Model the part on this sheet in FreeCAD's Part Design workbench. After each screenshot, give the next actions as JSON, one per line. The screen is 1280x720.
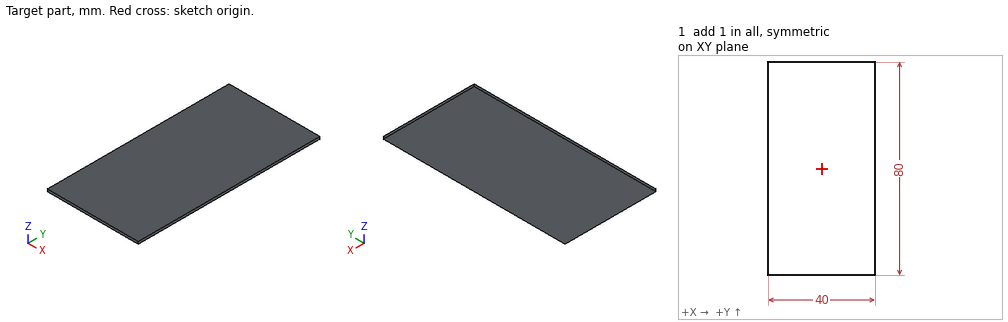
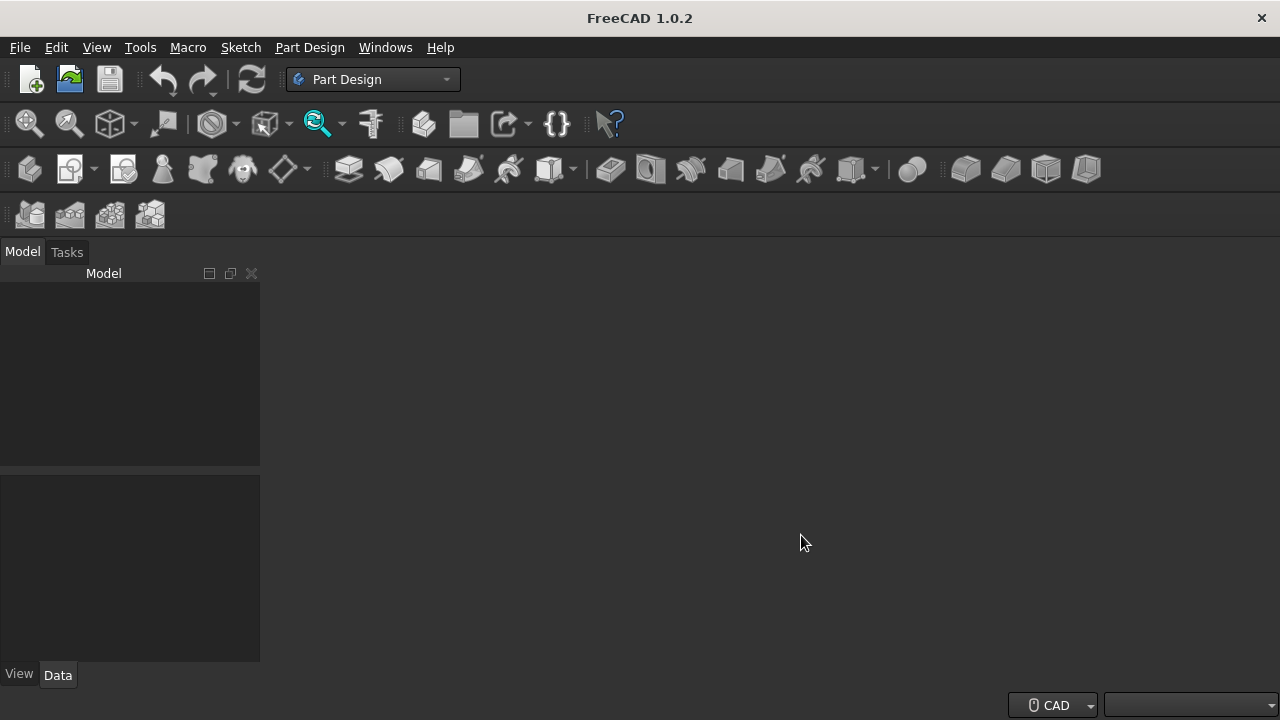
{"action": "left_click", "coordinate": [30, 80]}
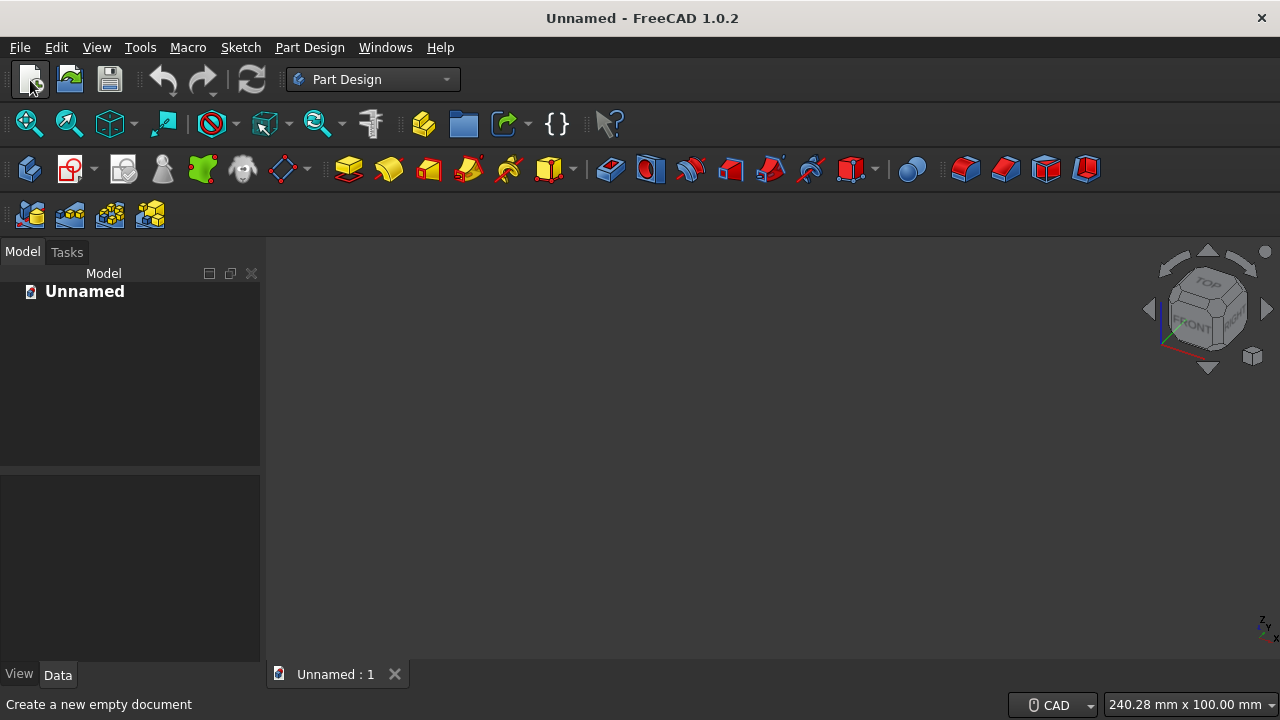
{"action": "left_click", "coordinate": [70, 170]}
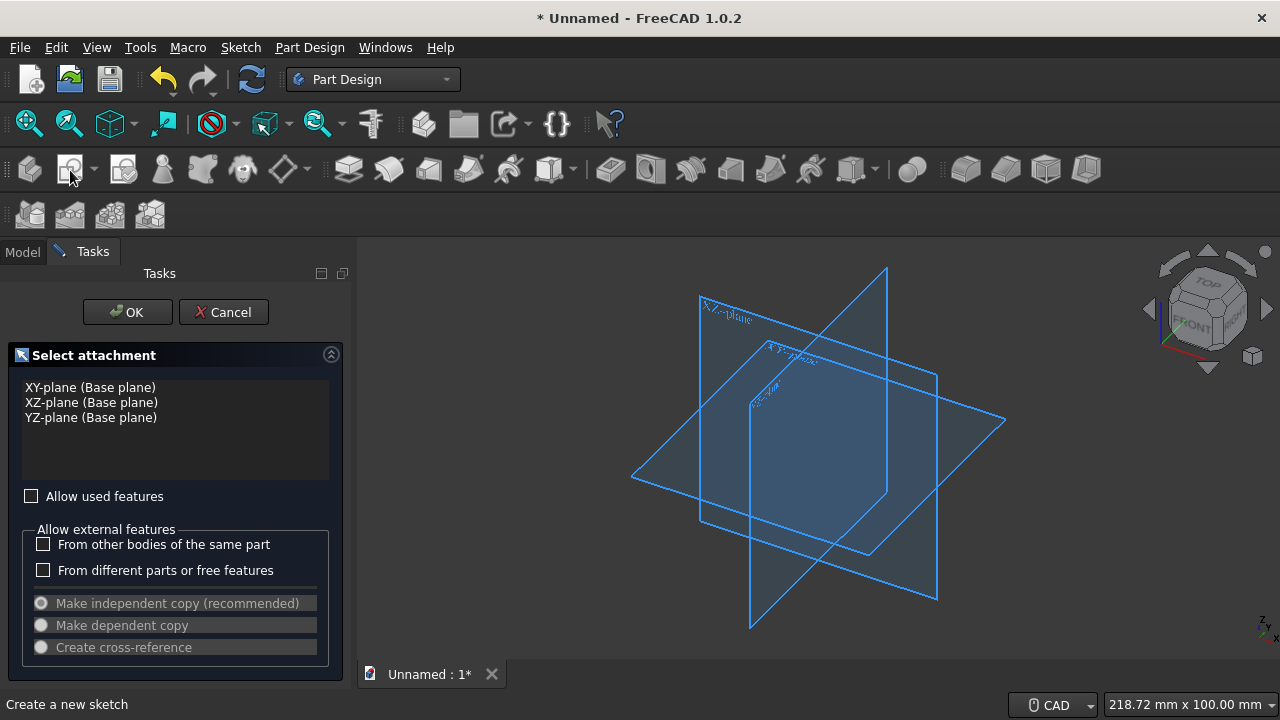
{"action": "left_click", "coordinate": [82, 388]}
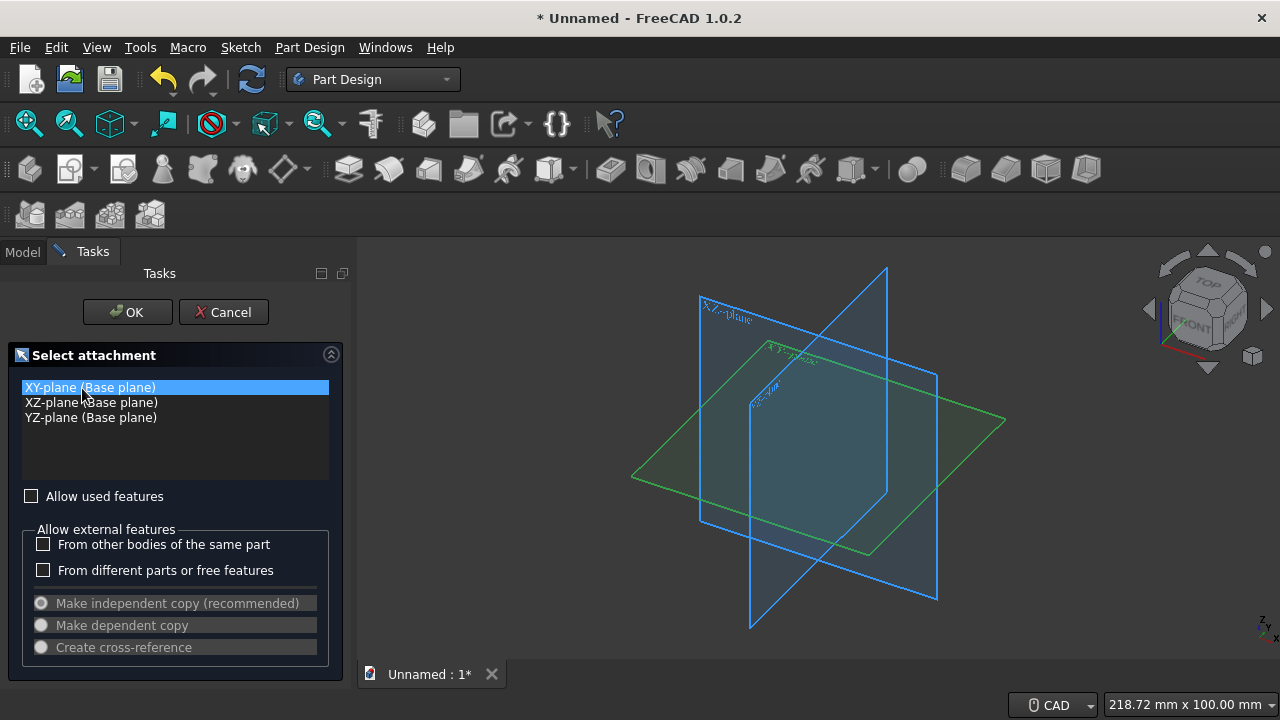
{"action": "left_click", "coordinate": [128, 312]}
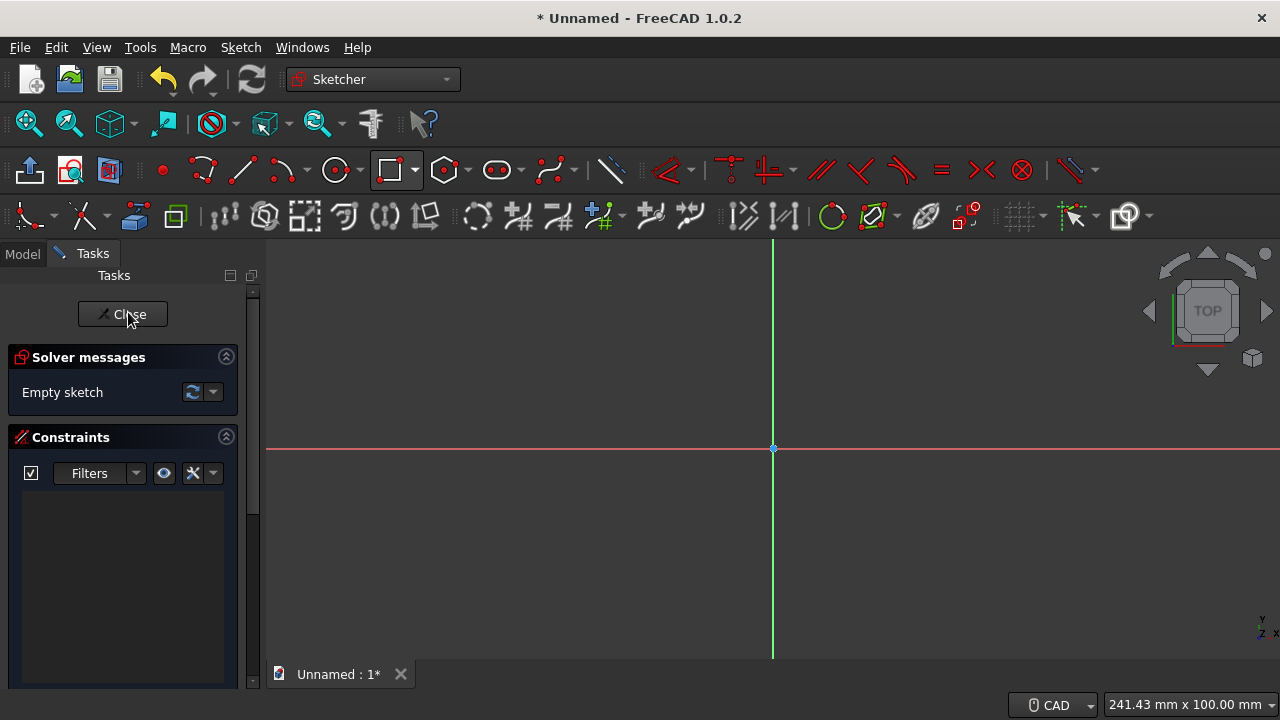
{"action": "scroll", "coordinate": [395, 449], "scroll_direction": "down", "scroll_amount": 1}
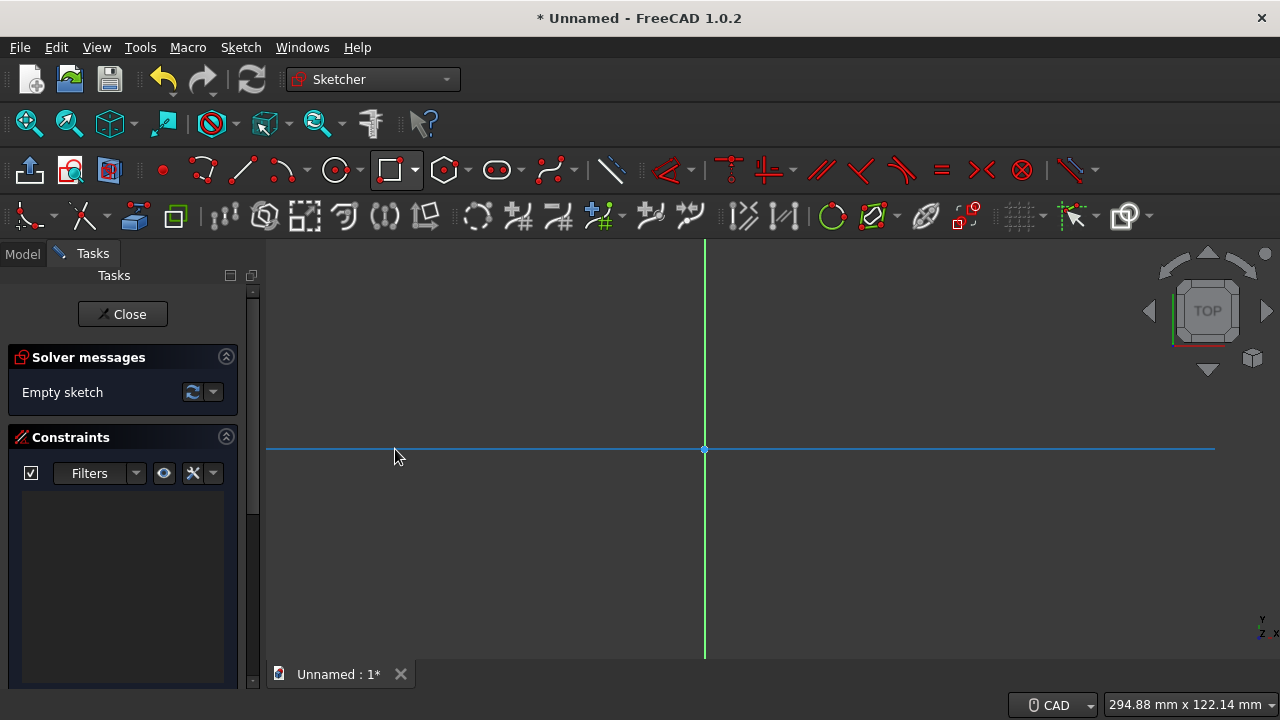
{"action": "left_click", "coordinate": [418, 170]}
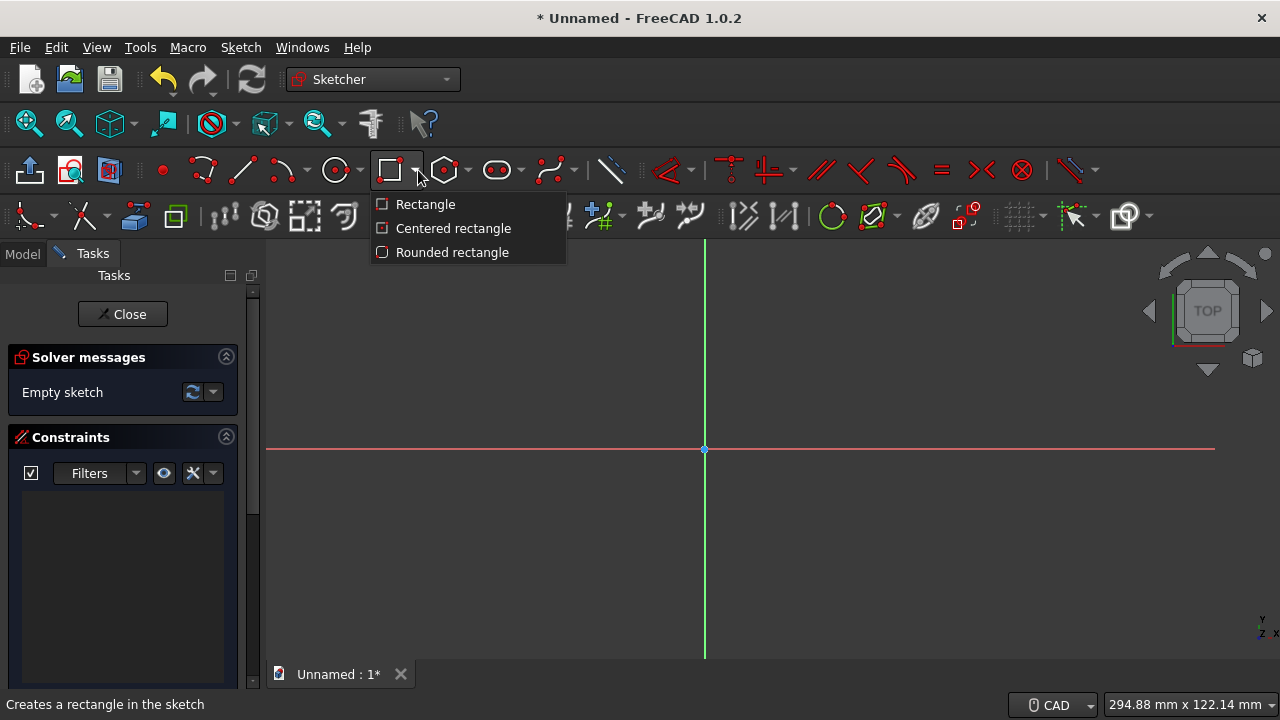
{"action": "left_click", "coordinate": [468, 228]}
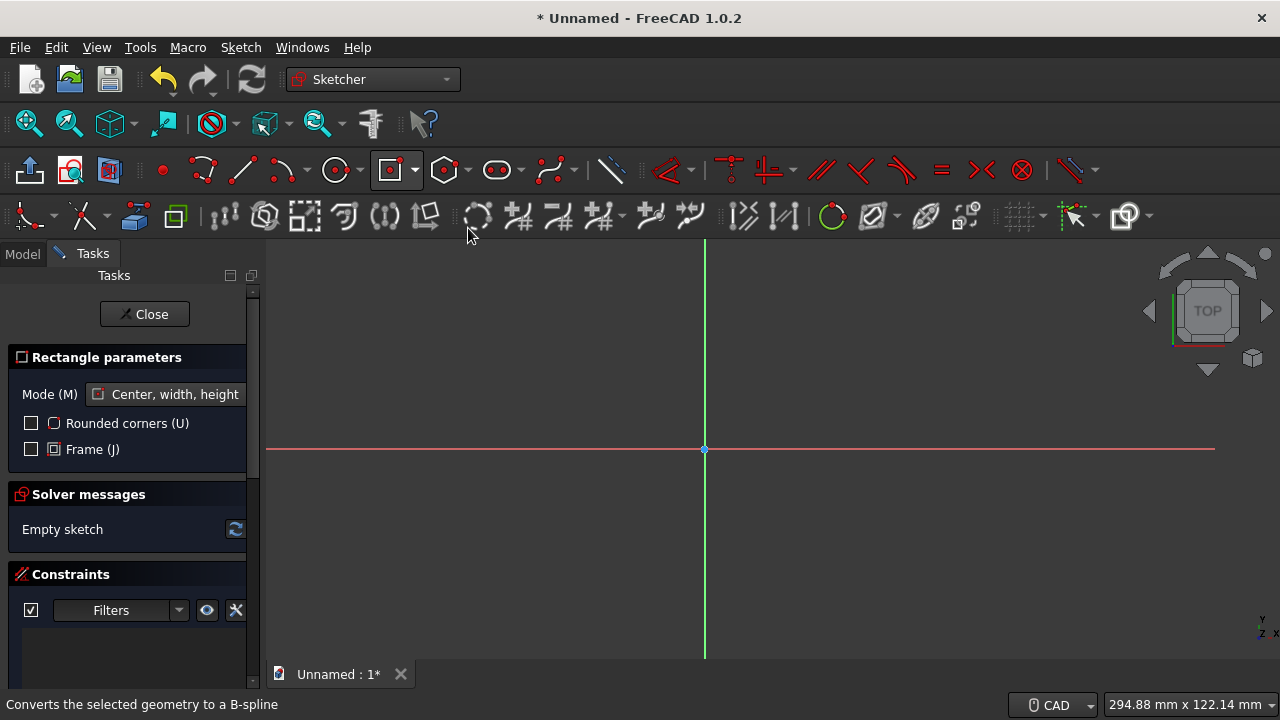
{"action": "left_click", "coordinate": [705, 449]}
{"action": "mouse_move", "coordinate": [773, 312]}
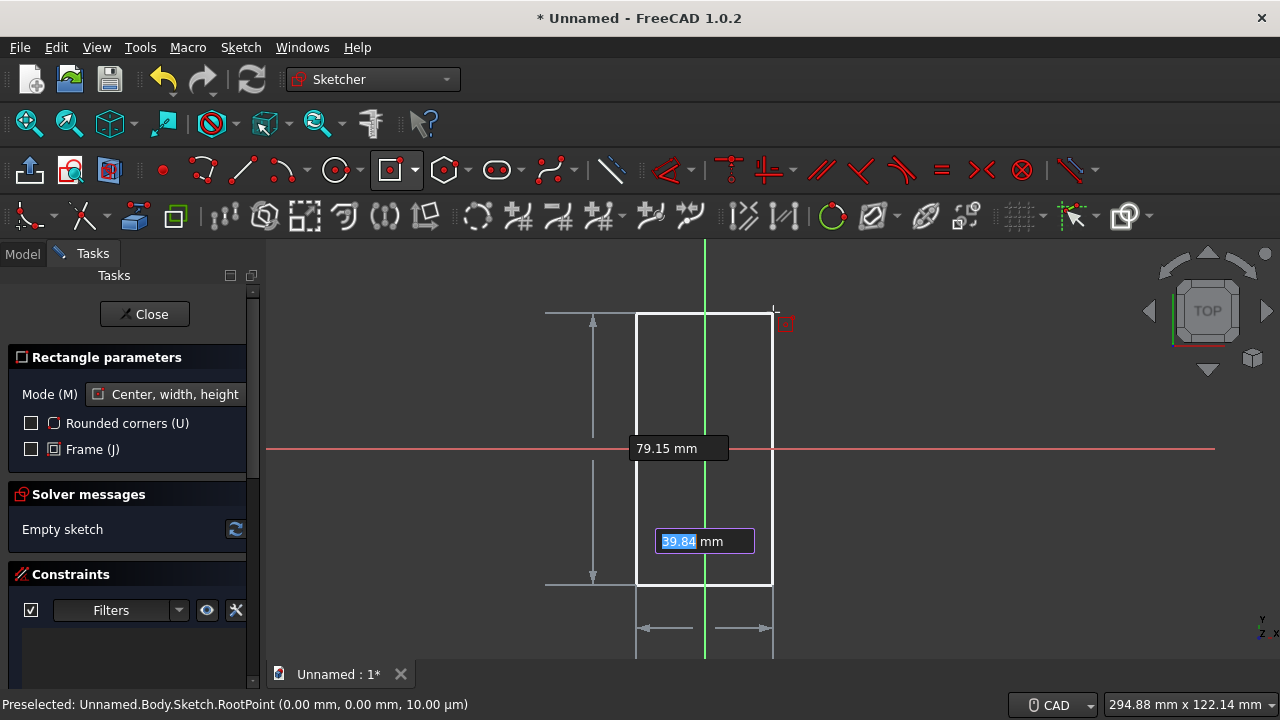
{"action": "type", "text": "40"}
{"action": "key", "text": "Tab"}
{"action": "type", "text": "80"}
{"action": "key", "text": "Return"}
{"action": "key", "text": "Escape"}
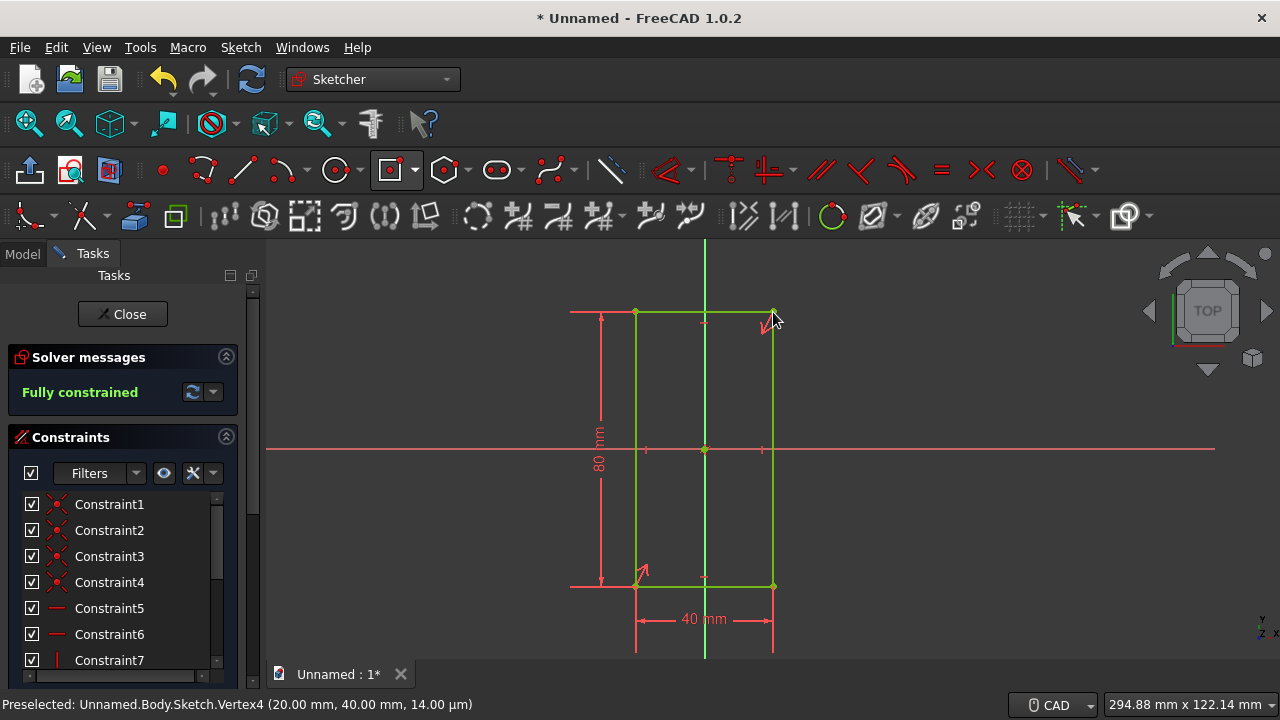
{"action": "left_click", "coordinate": [123, 314]}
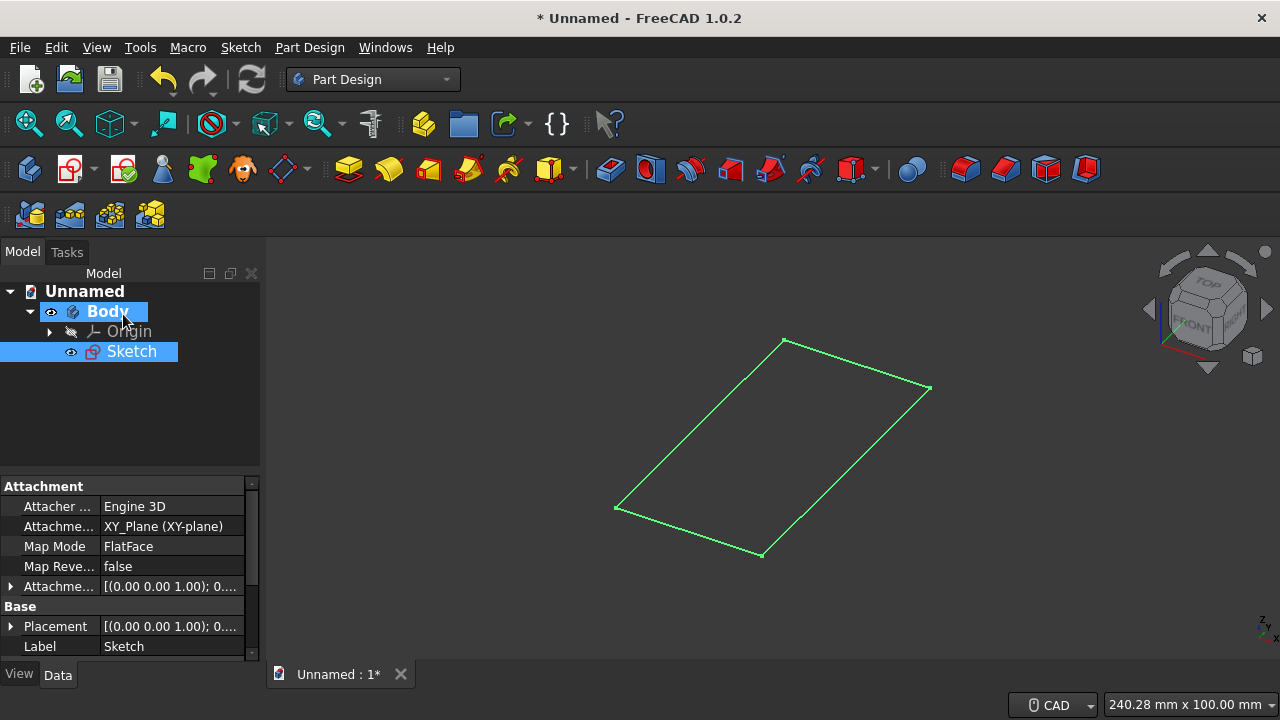
{"action": "left_click", "coordinate": [350, 170]}